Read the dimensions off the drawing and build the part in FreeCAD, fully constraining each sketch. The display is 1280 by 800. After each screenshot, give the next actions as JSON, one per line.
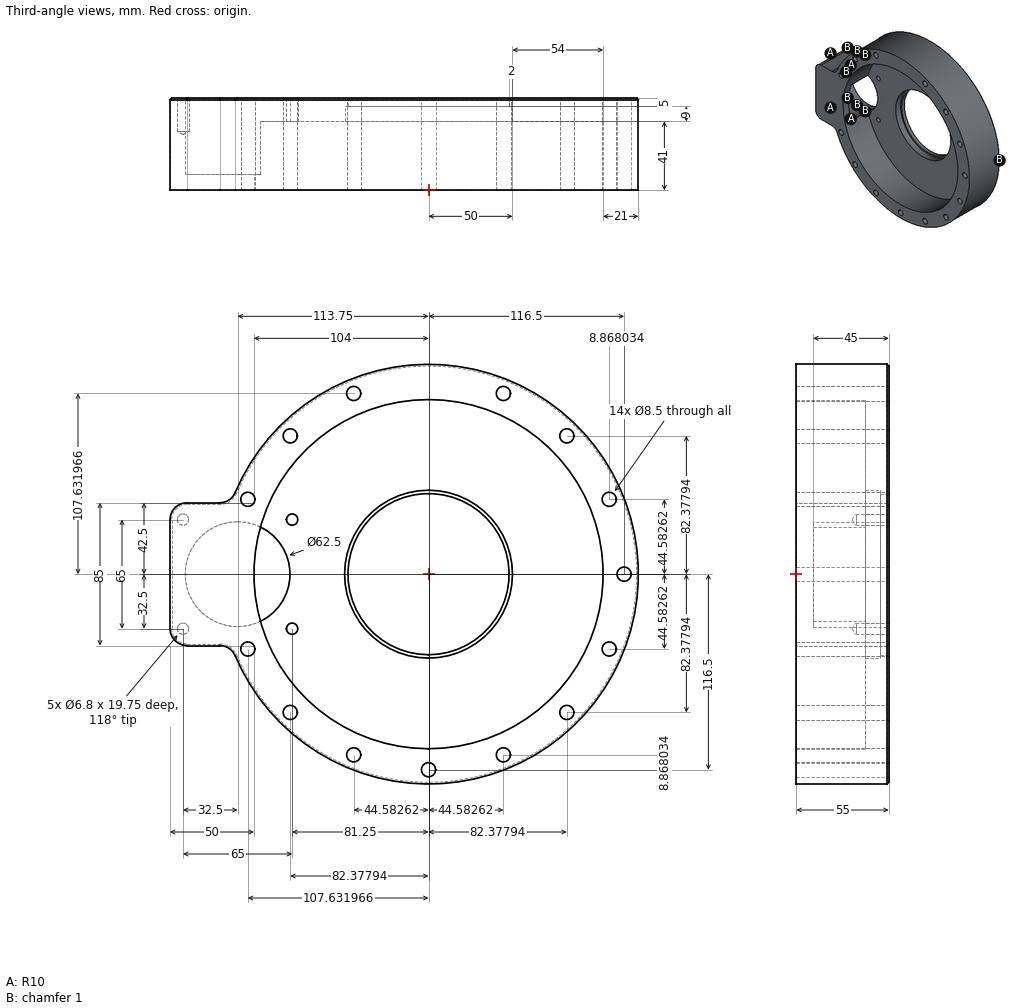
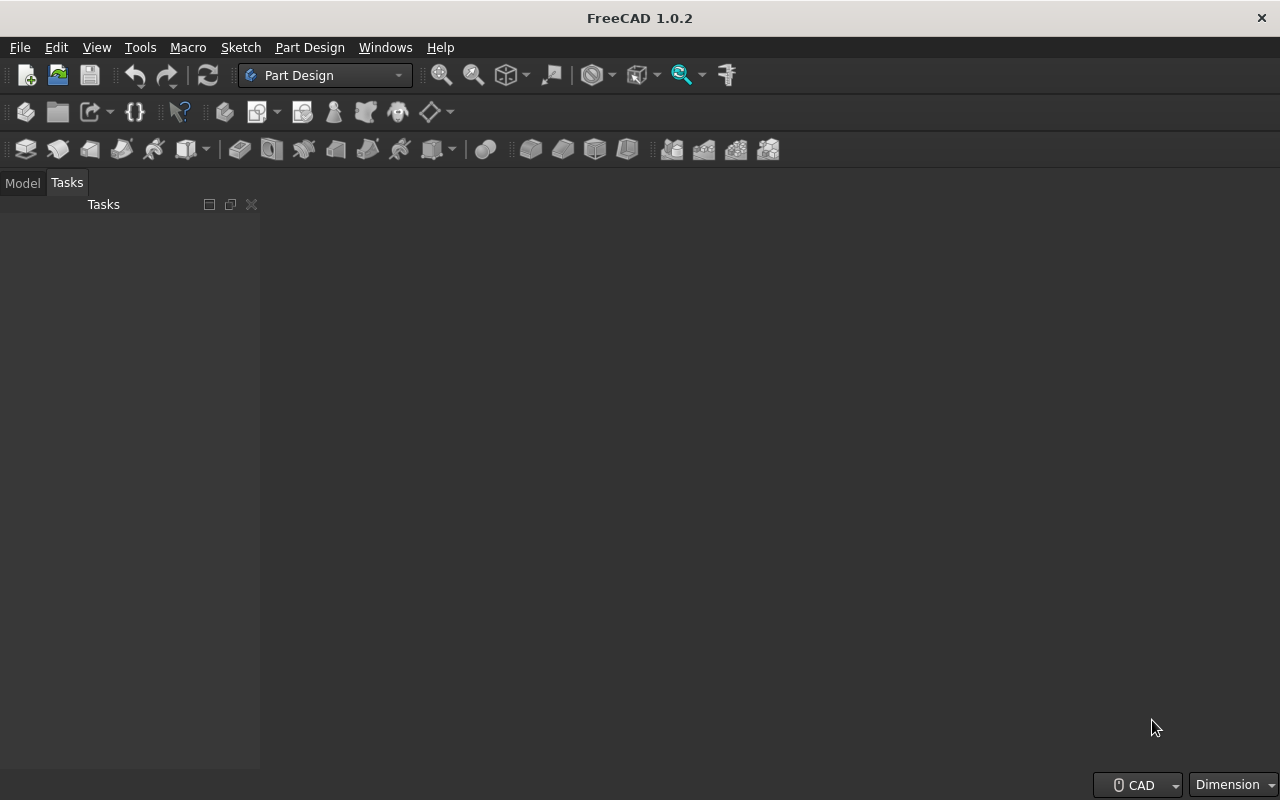
{"action": "left_click", "coordinate": [26, 76]}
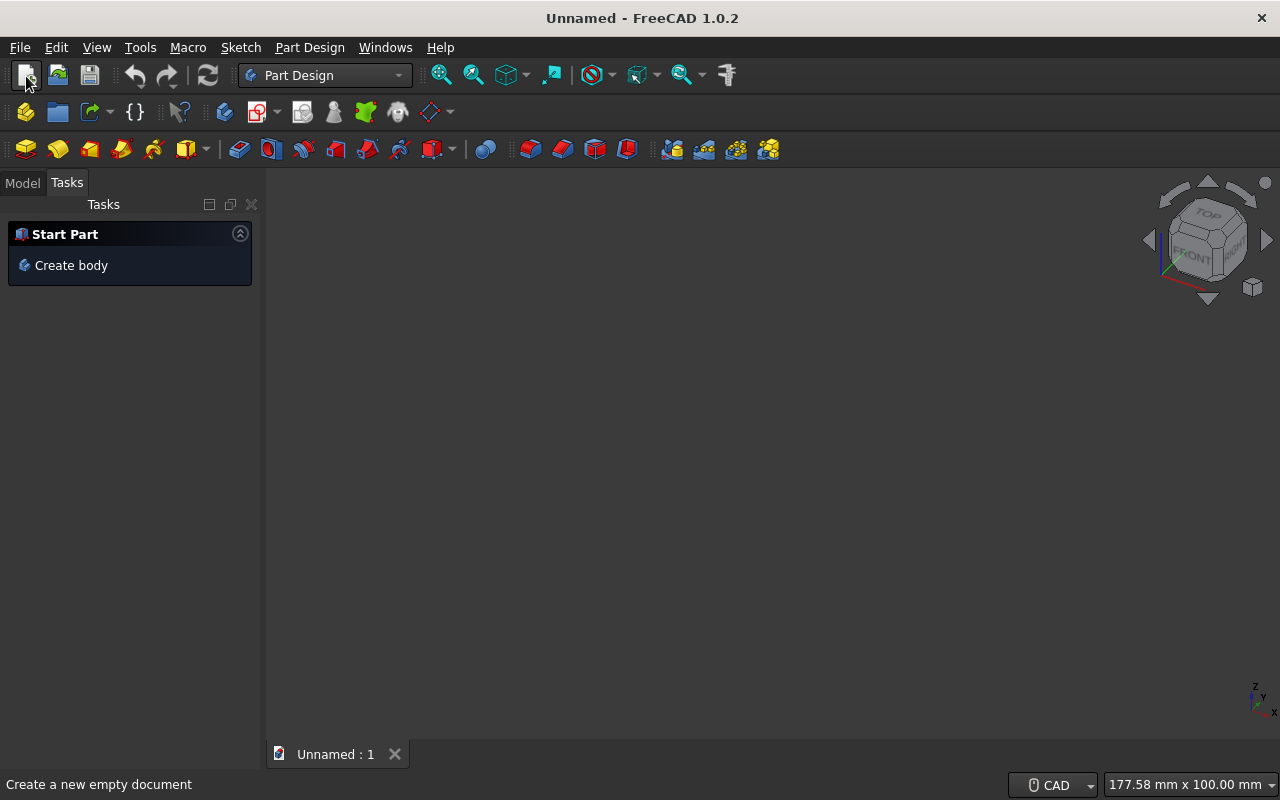
{"action": "left_click", "coordinate": [258, 112]}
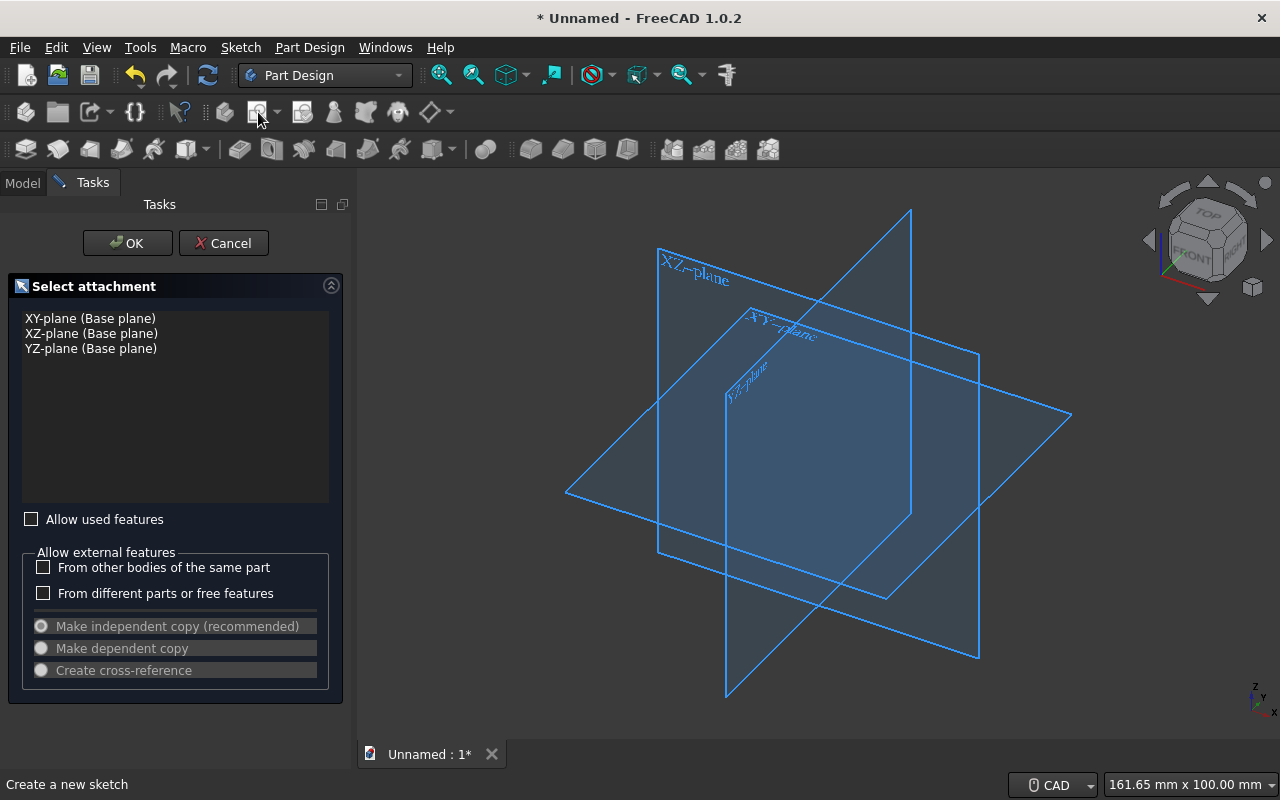
{"action": "left_click", "coordinate": [82, 318]}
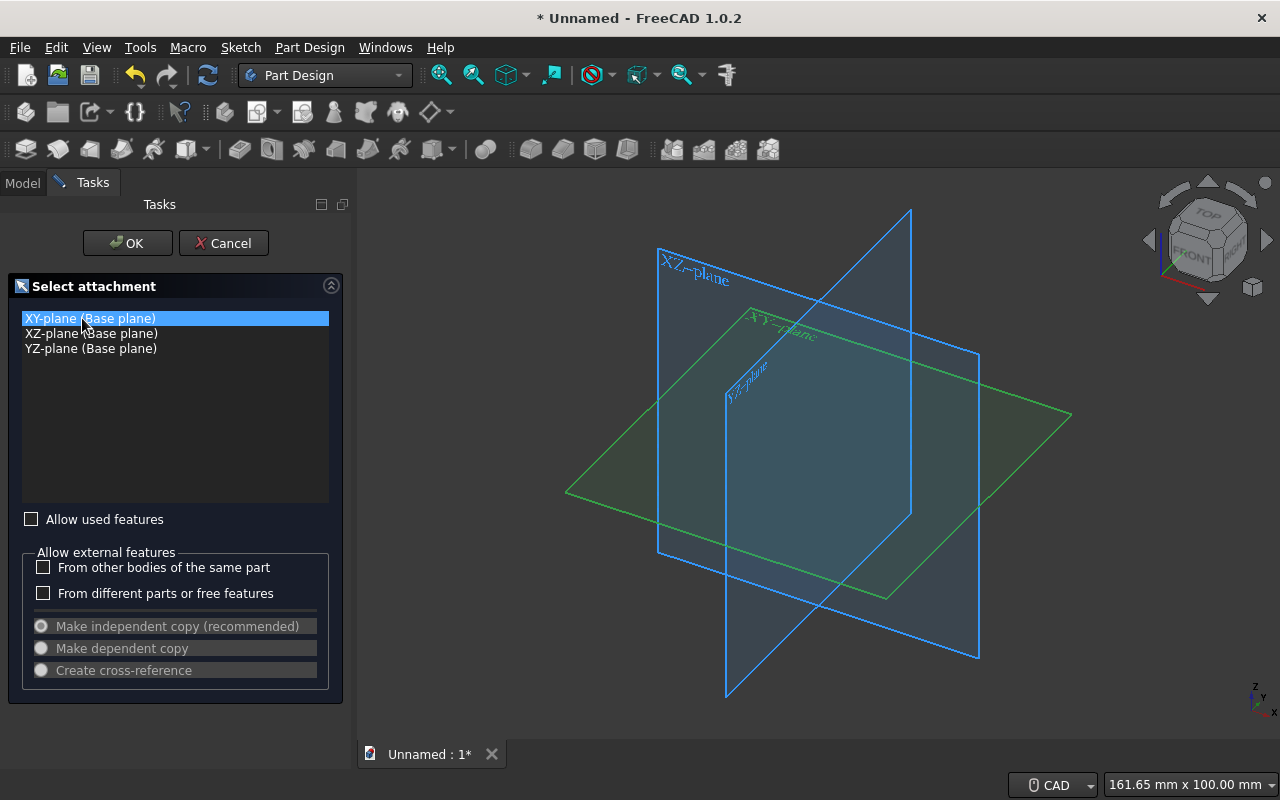
{"action": "left_click", "coordinate": [128, 243]}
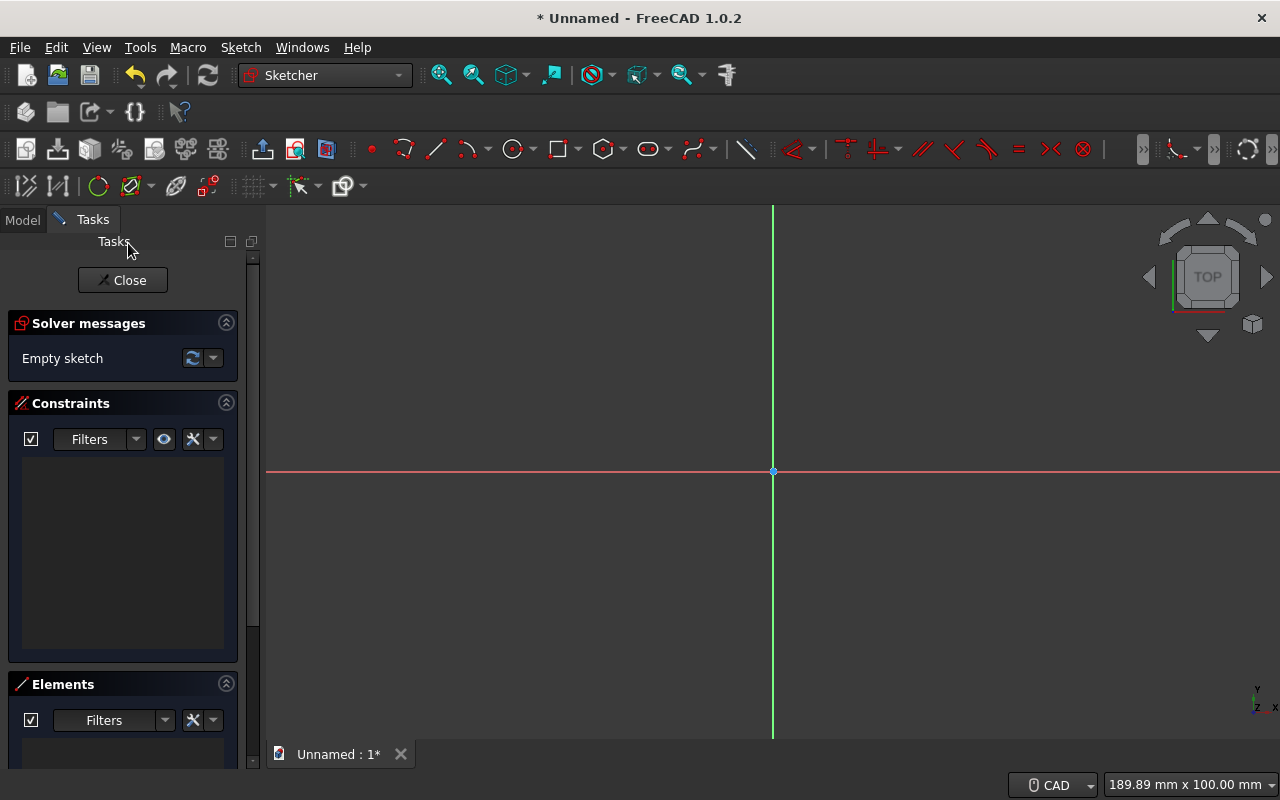
{"action": "scroll", "coordinate": [294, 711], "scroll_direction": "down", "scroll_amount": 2}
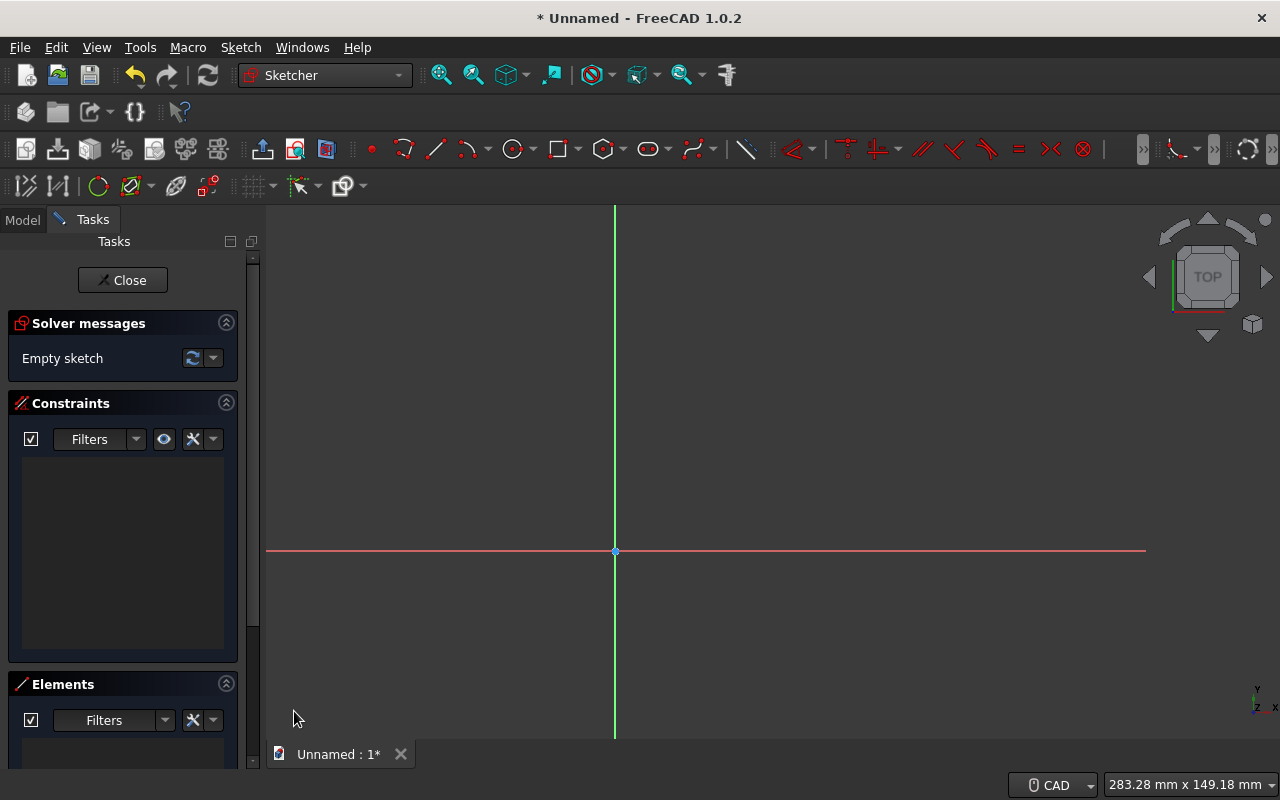
{"action": "left_click", "coordinate": [404, 150]}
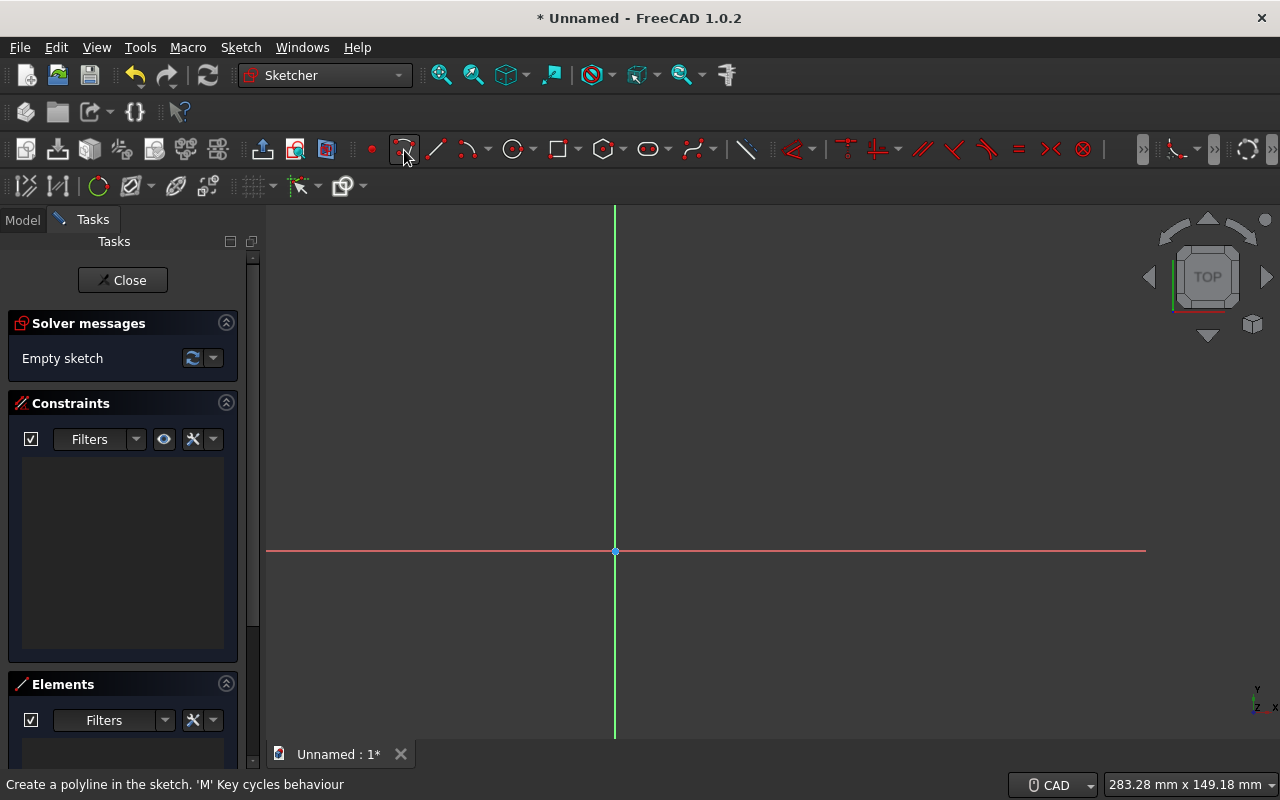
{"action": "left_click", "coordinate": [794, 404]}
{"action": "left_click", "coordinate": [987, 404]}
{"action": "left_click", "coordinate": [987, 551]}
{"action": "left_click", "coordinate": [1063, 542]}
{"action": "left_click", "coordinate": [1063, 354]}
{"action": "left_click", "coordinate": [787, 354]}
{"action": "left_click", "coordinate": [787, 372]}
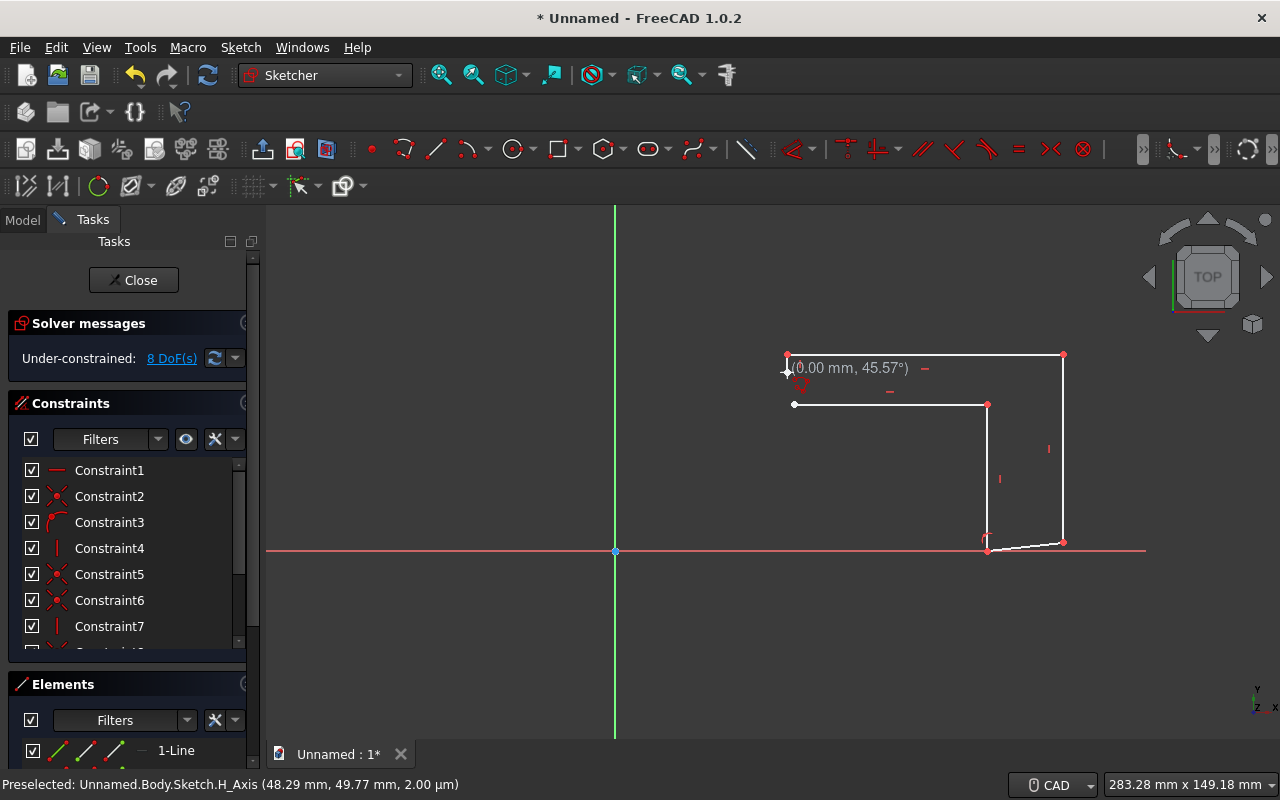
{"action": "scroll", "coordinate": [794, 372], "scroll_direction": "up", "scroll_amount": 4}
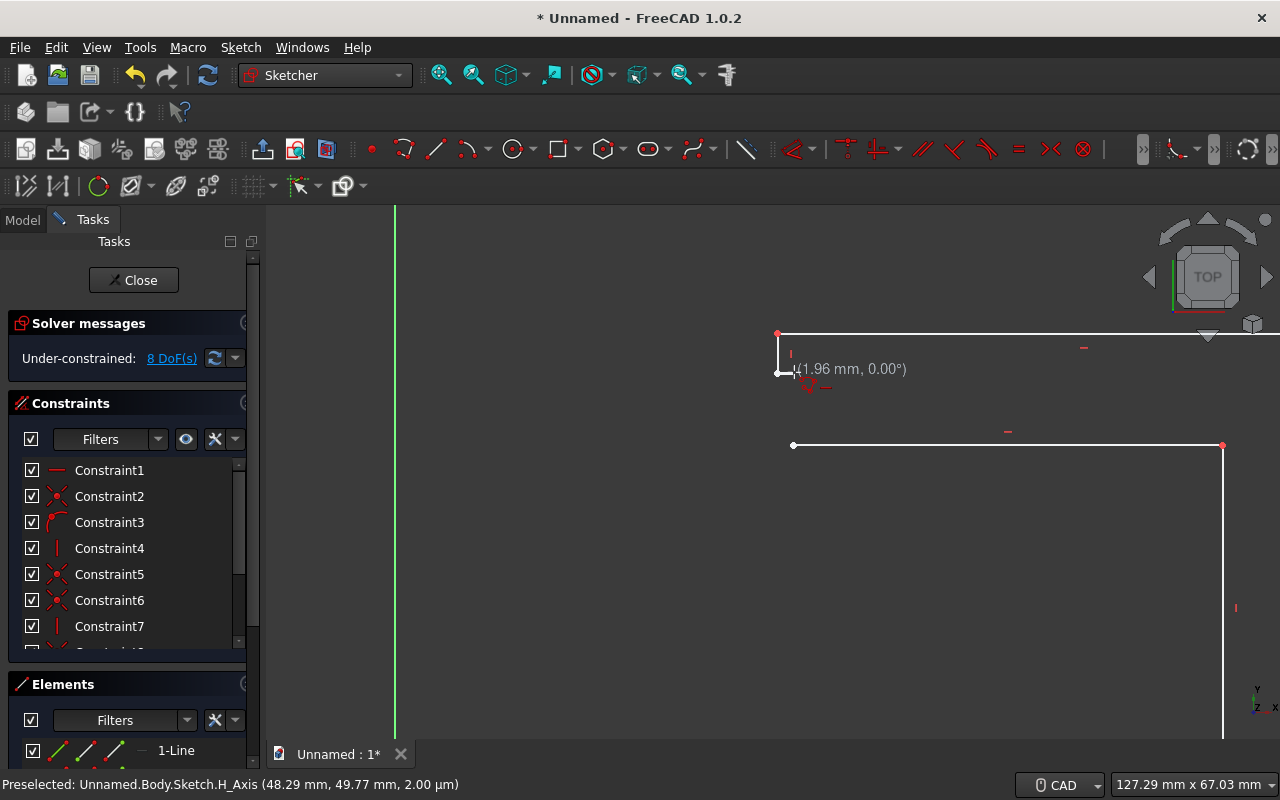
{"action": "left_click", "coordinate": [794, 372]}
{"action": "left_click", "coordinate": [793, 445]}
{"action": "key", "text": "Escape"}
{"action": "key", "text": "Escape"}